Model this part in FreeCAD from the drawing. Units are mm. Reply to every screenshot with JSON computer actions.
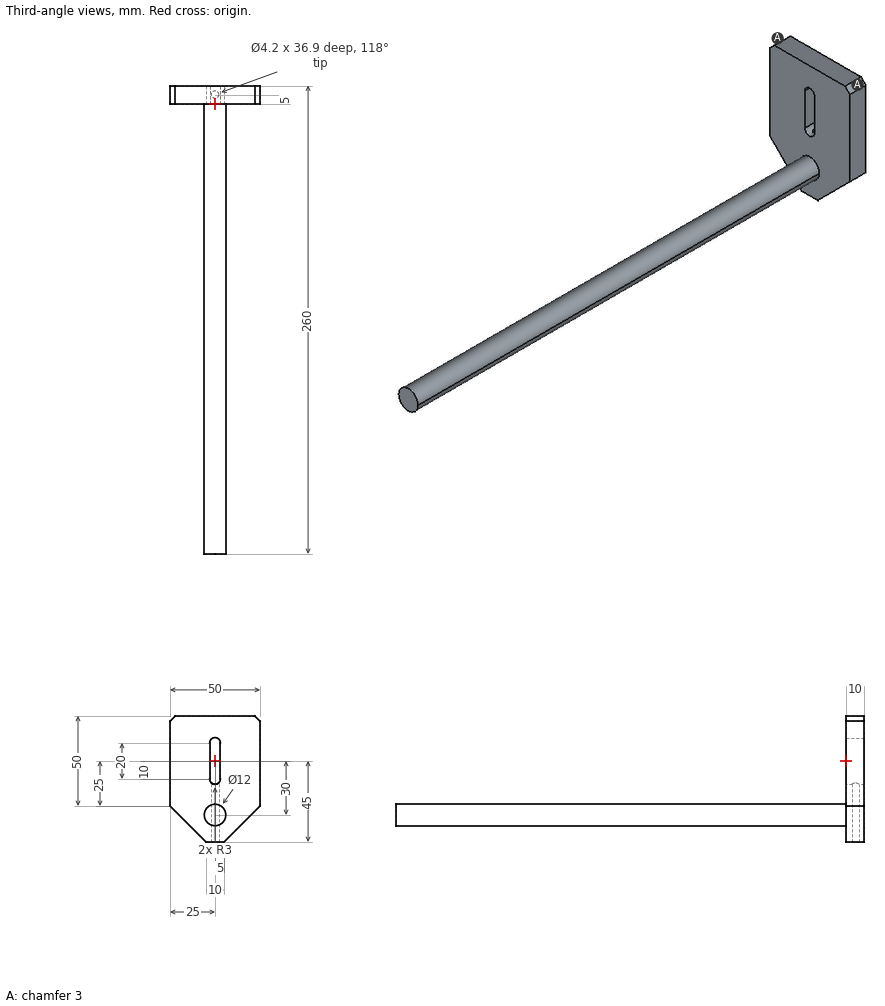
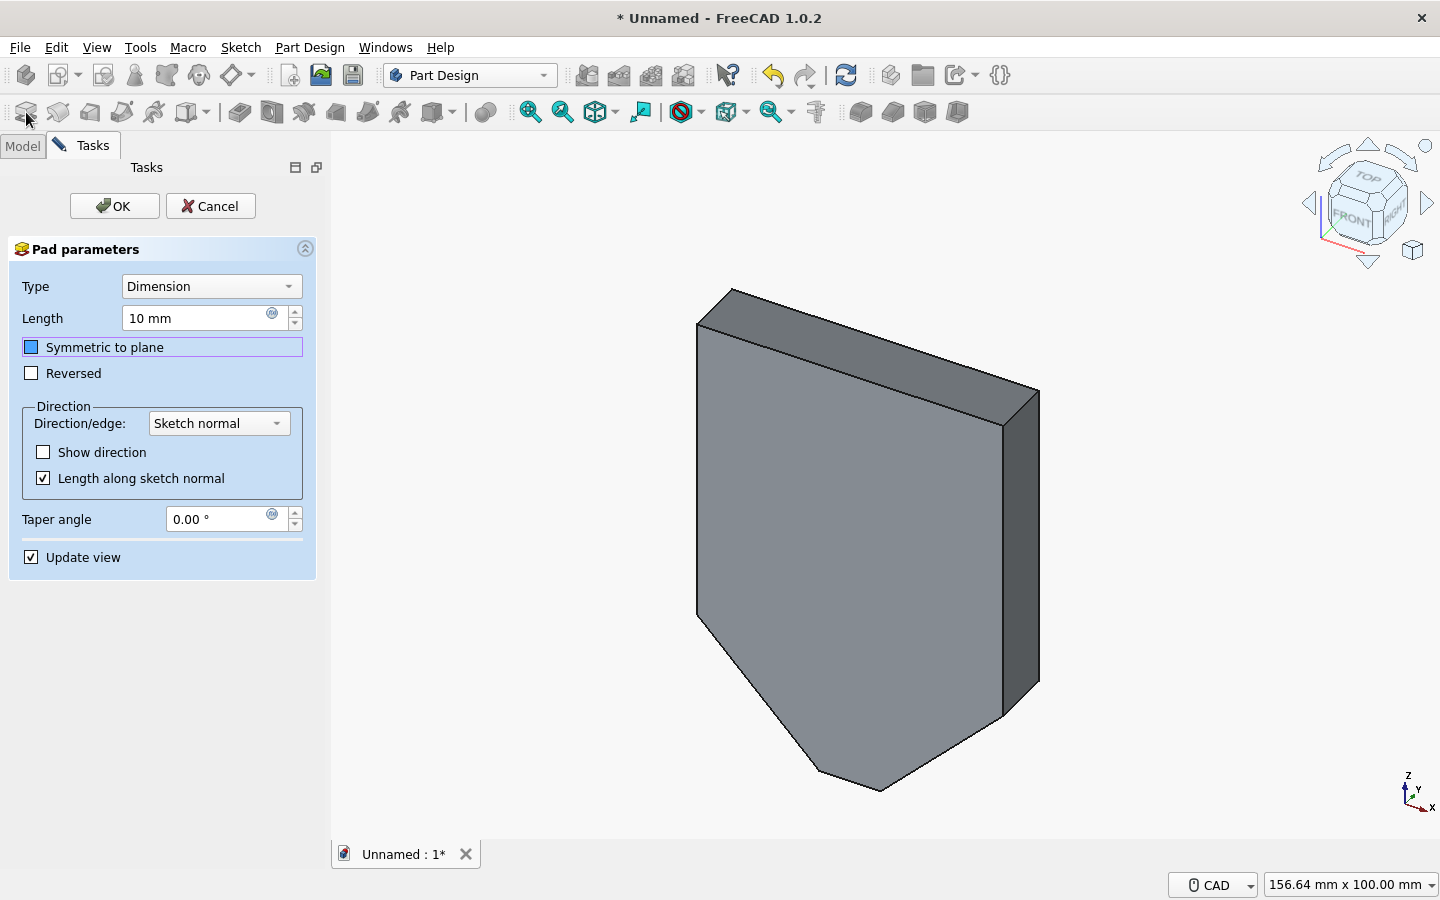
{"action": "left_click", "coordinate": [30, 373]}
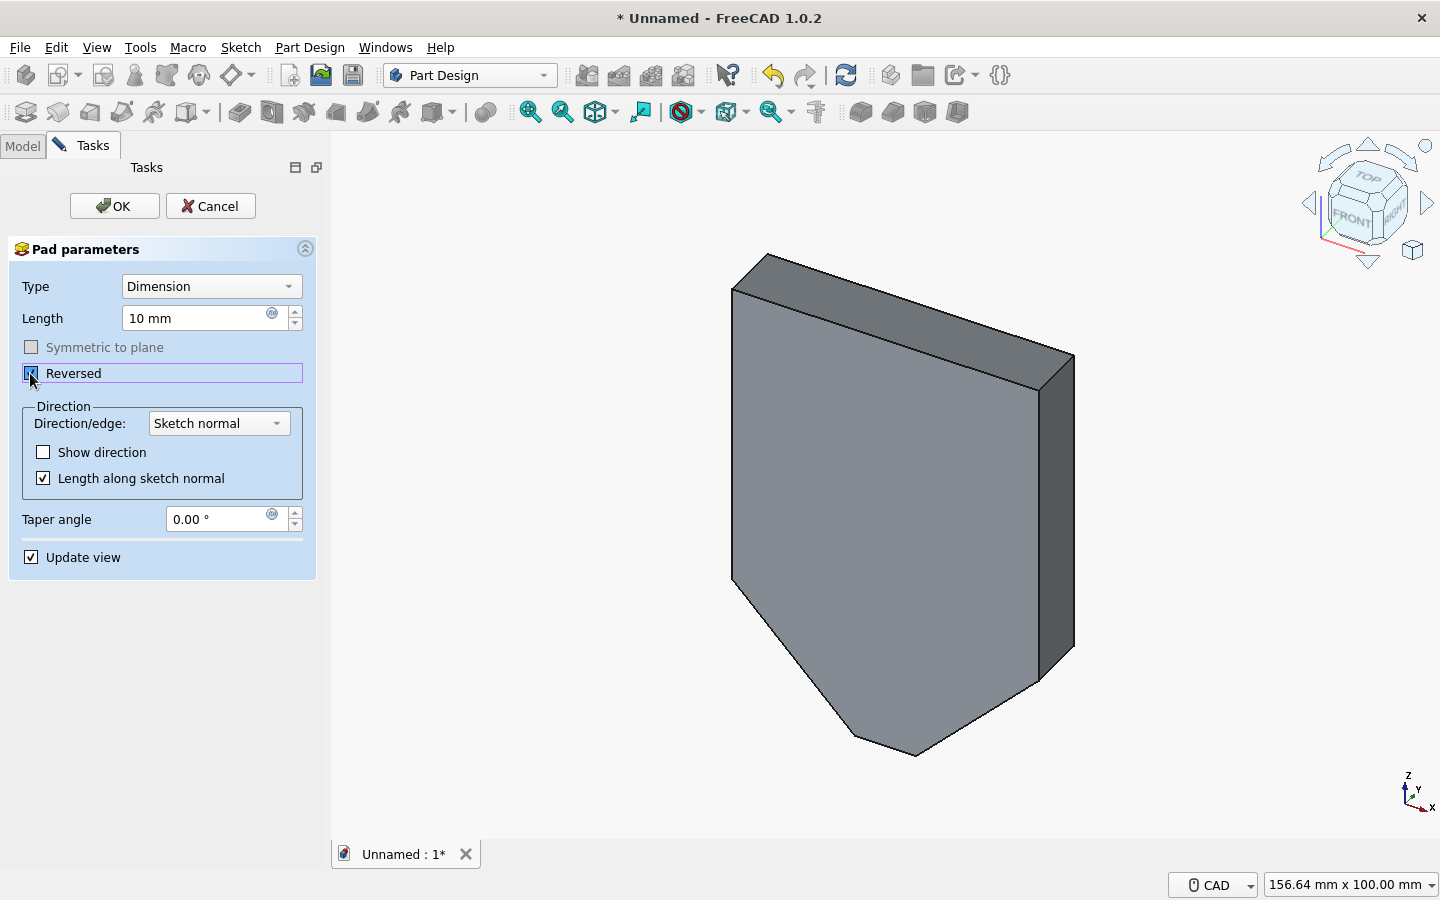
{"action": "left_click", "coordinate": [115, 206]}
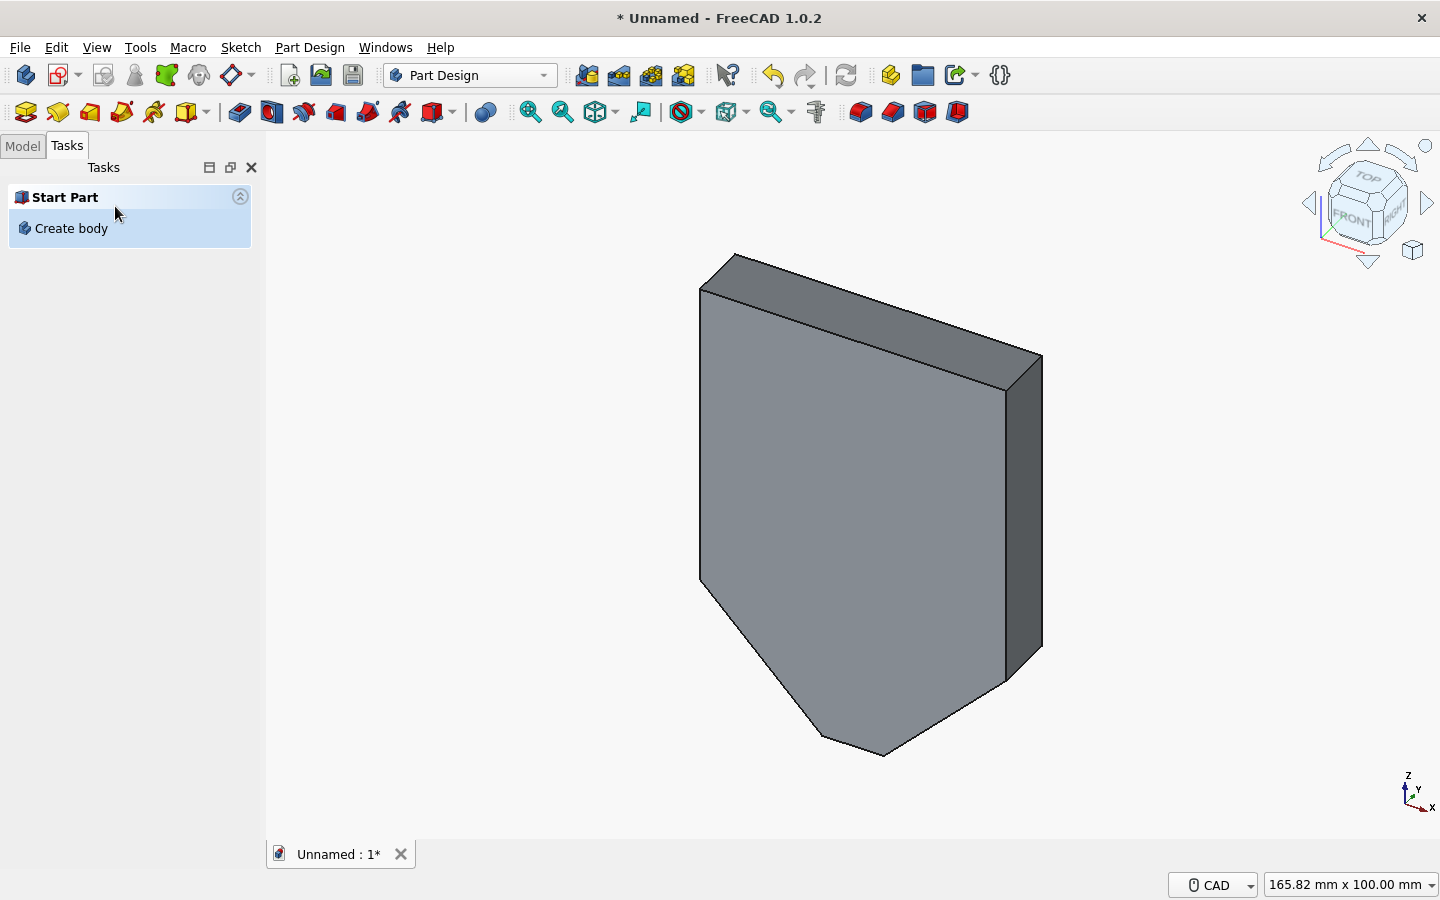
{"action": "key", "text": "4"}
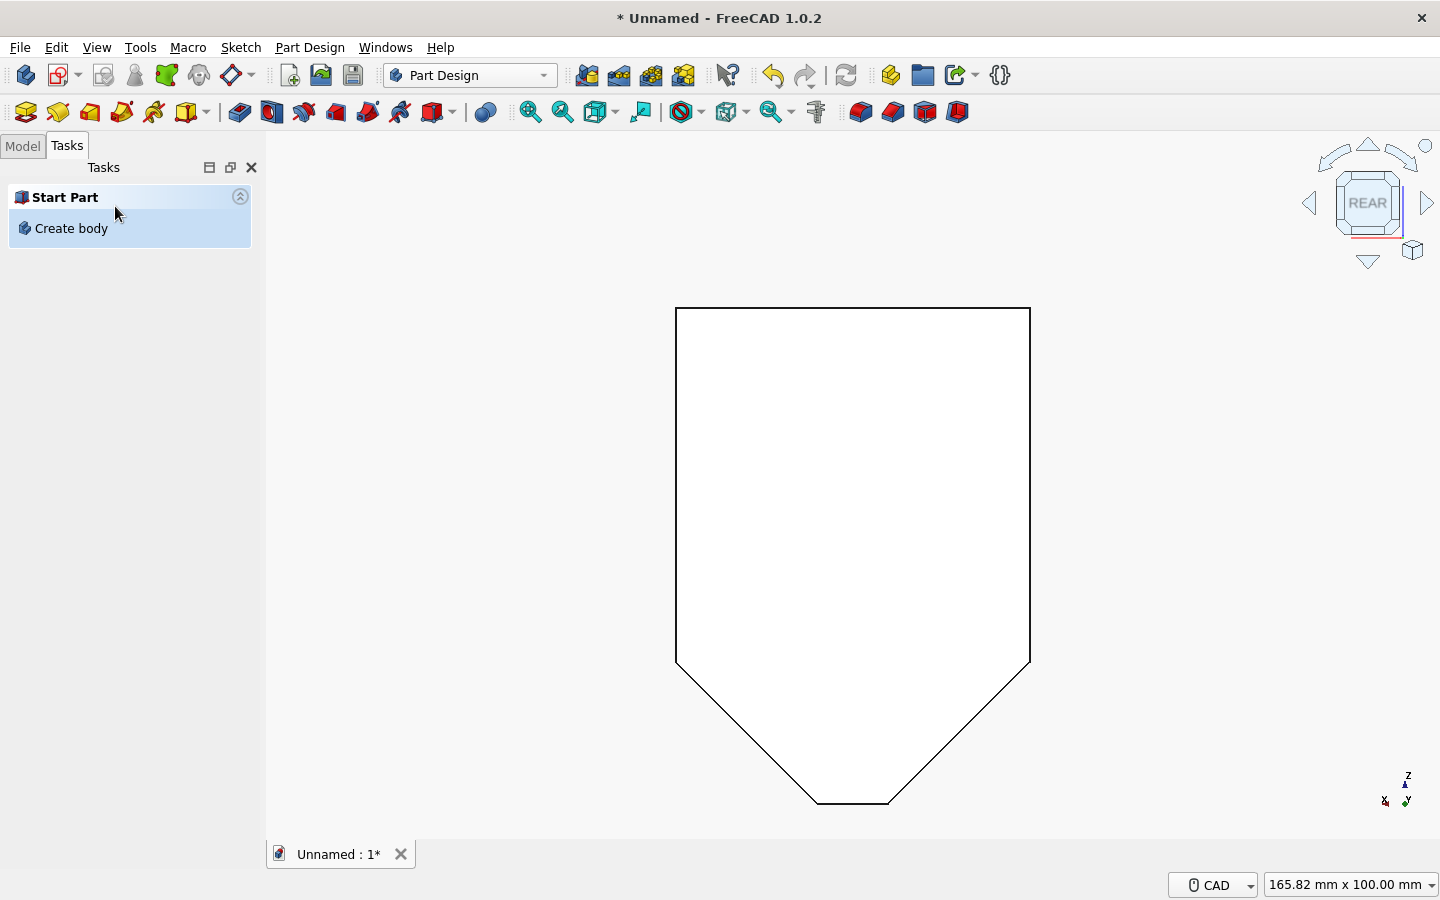
{"action": "left_click", "coordinate": [853, 484]}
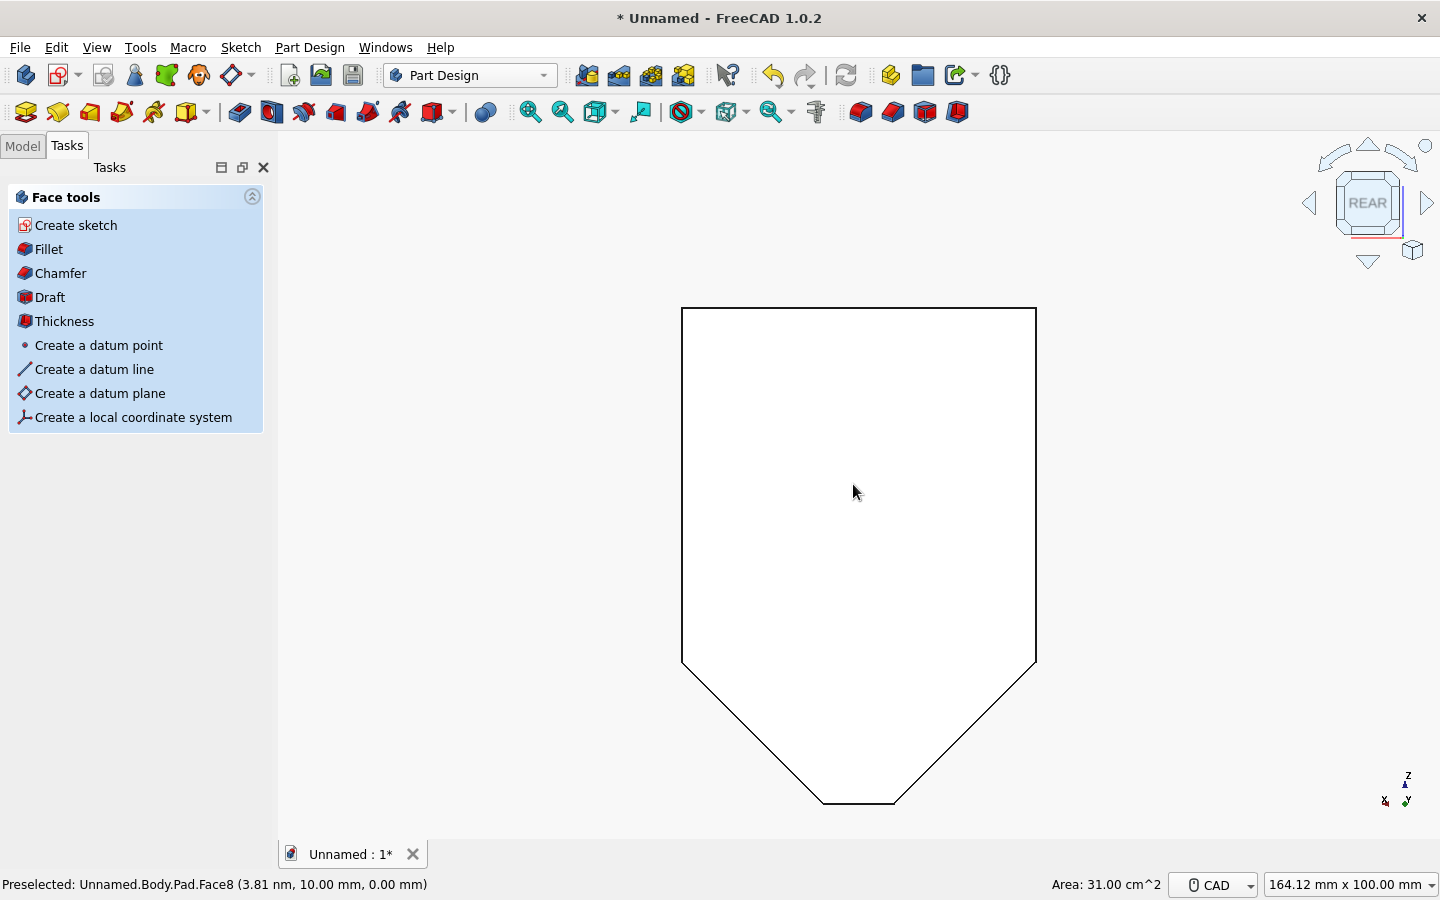
{"action": "left_click", "coordinate": [58, 76]}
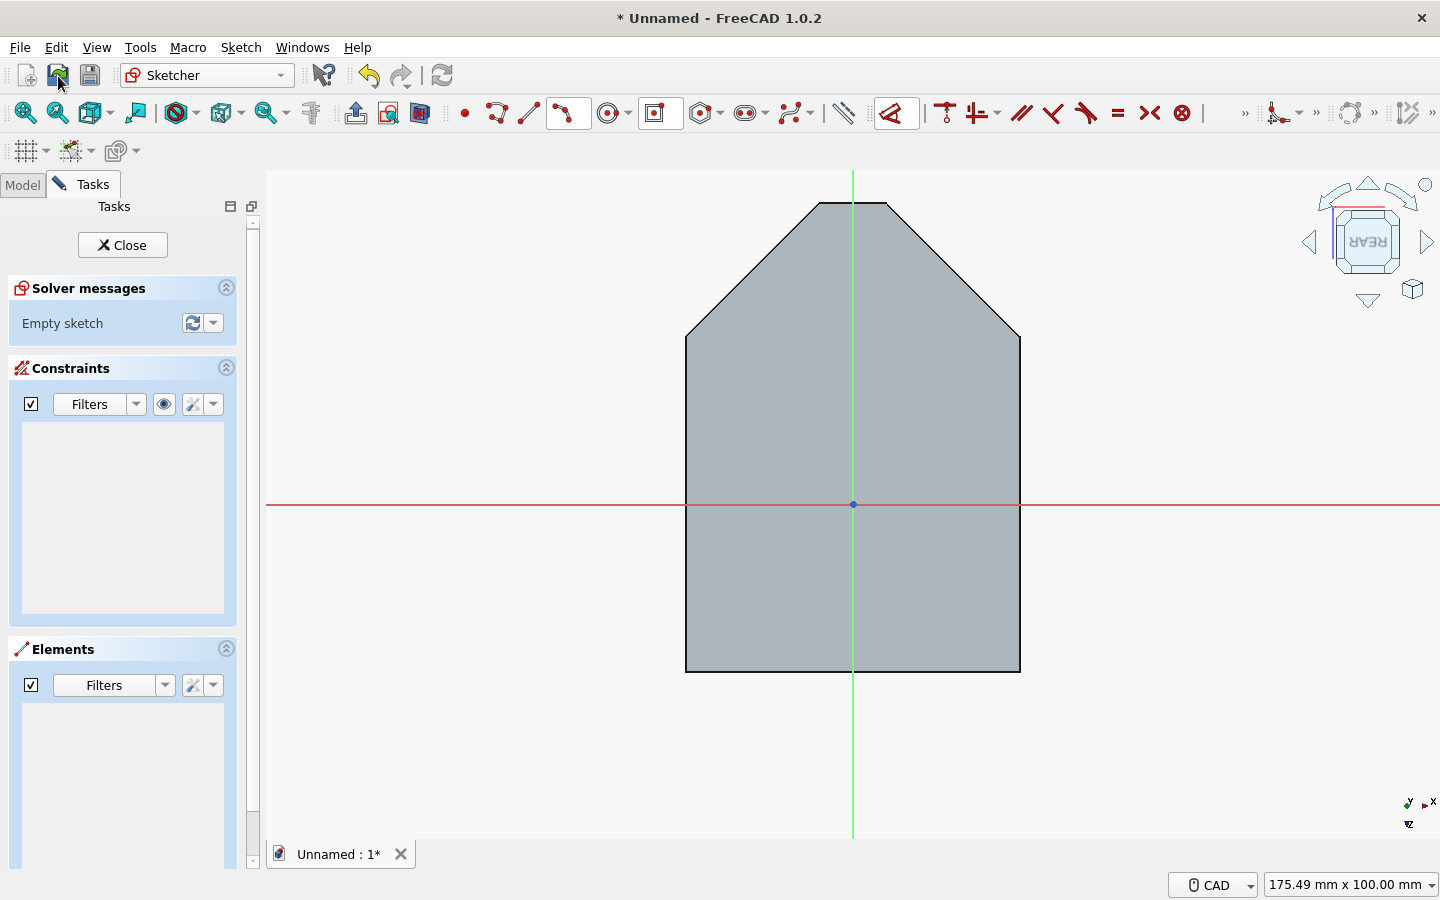
{"action": "scroll", "coordinate": [870, 253], "scroll_direction": "up", "scroll_amount": 8}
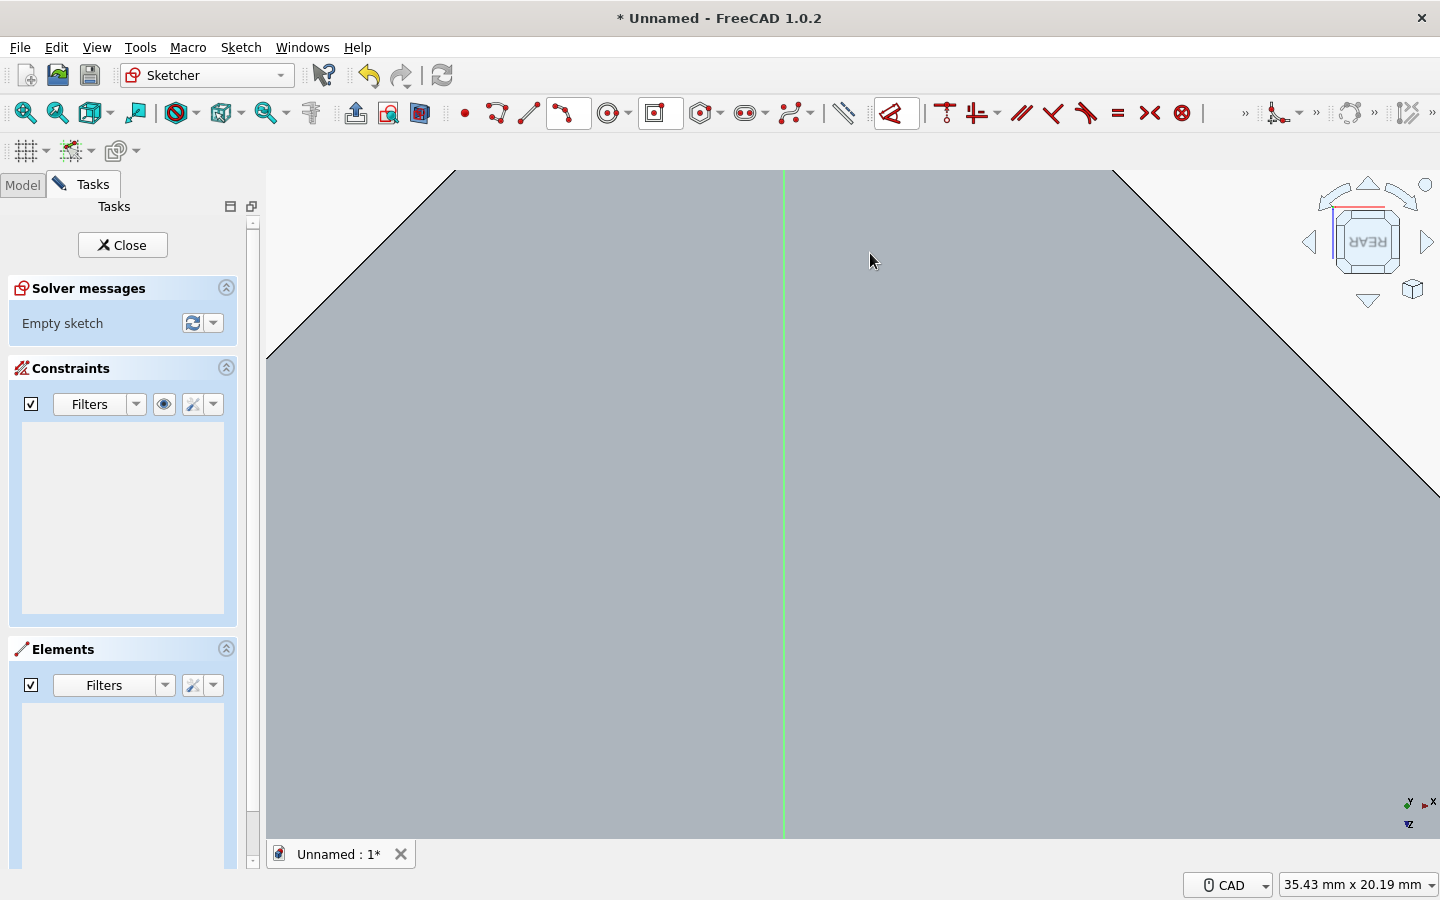
{"action": "left_click", "coordinate": [608, 114]}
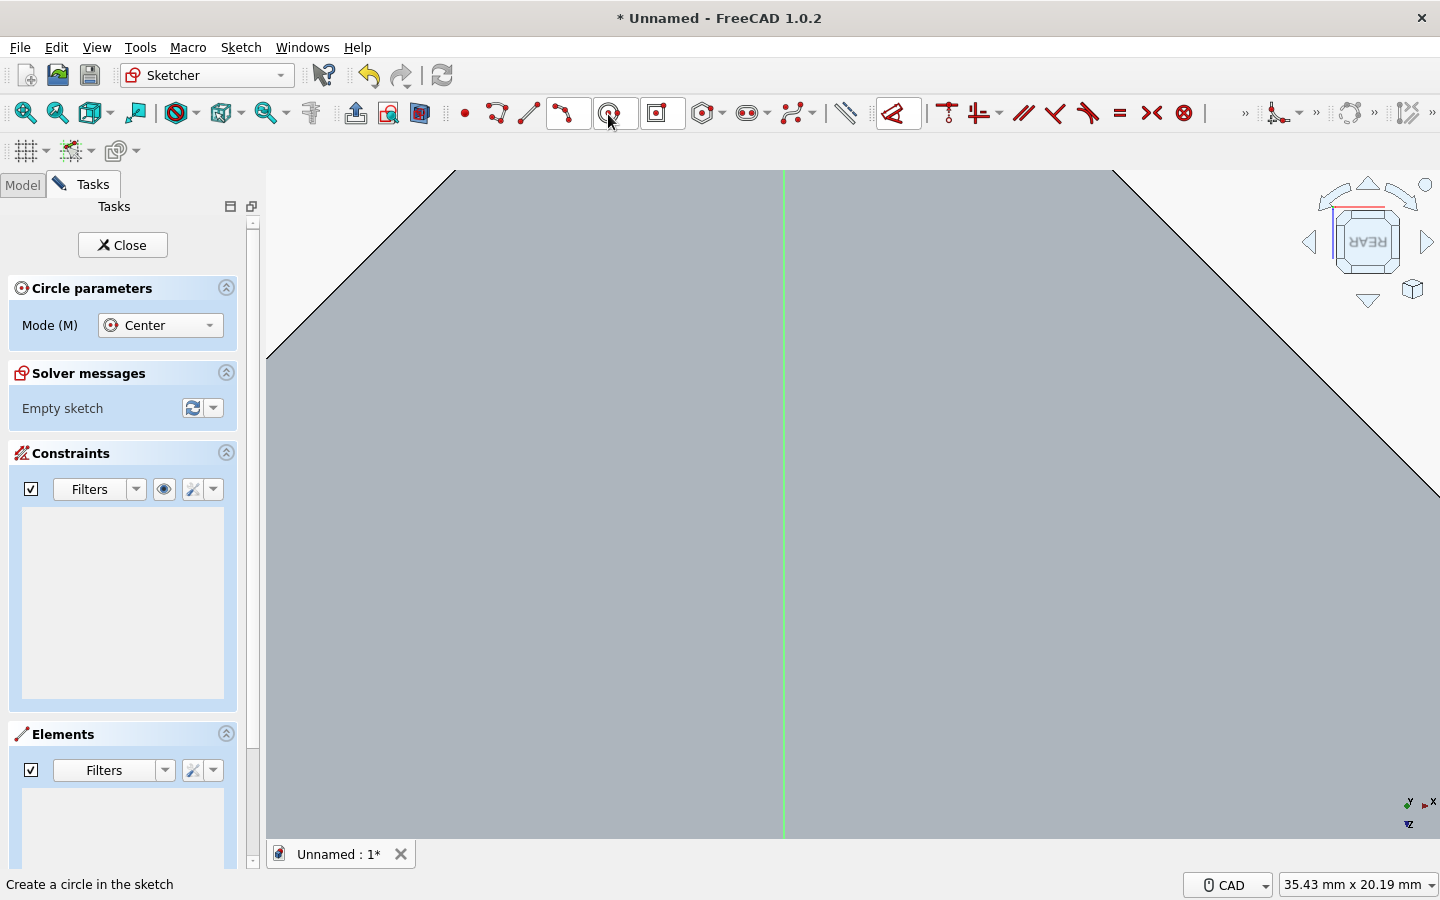
{"action": "left_click", "coordinate": [784, 504]}
{"action": "mouse_move", "coordinate": [924, 364]}